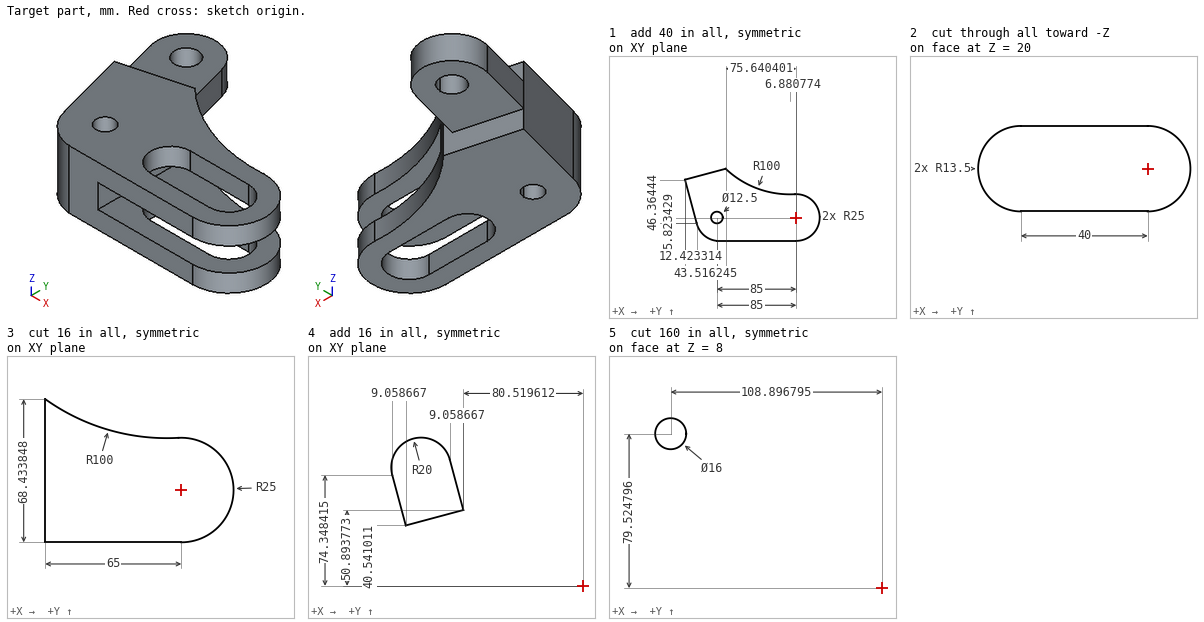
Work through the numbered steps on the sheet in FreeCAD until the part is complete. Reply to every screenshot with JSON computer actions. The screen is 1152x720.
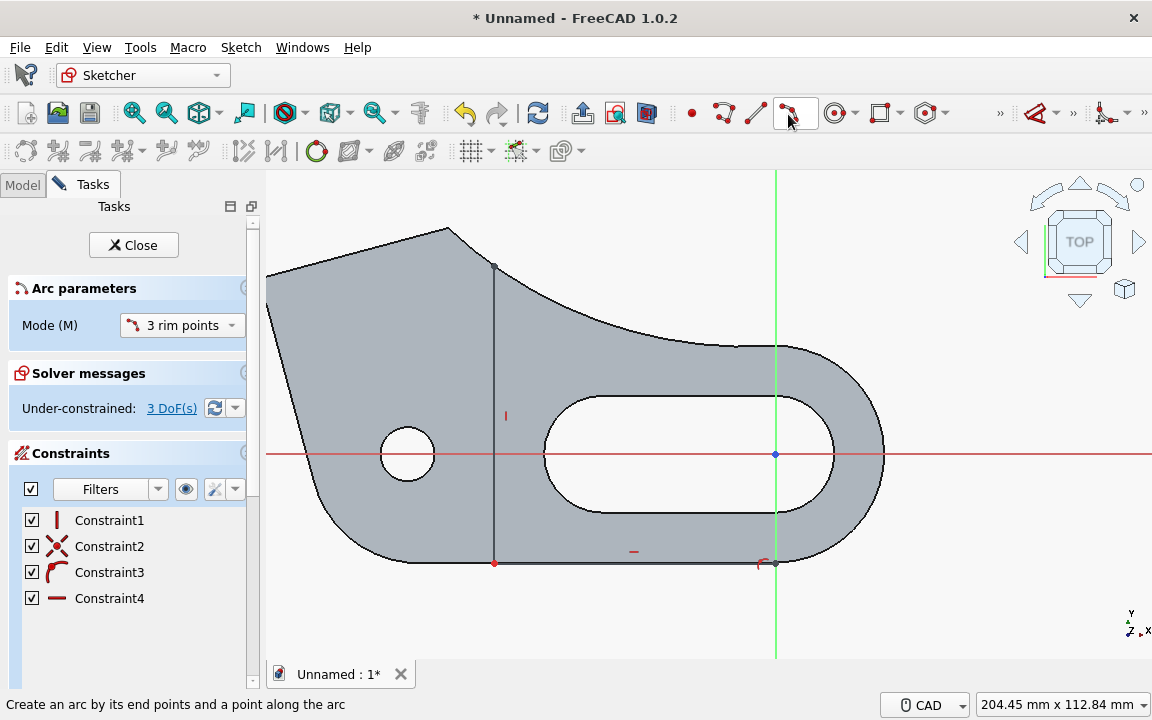
{"action": "left_click", "coordinate": [776, 564]}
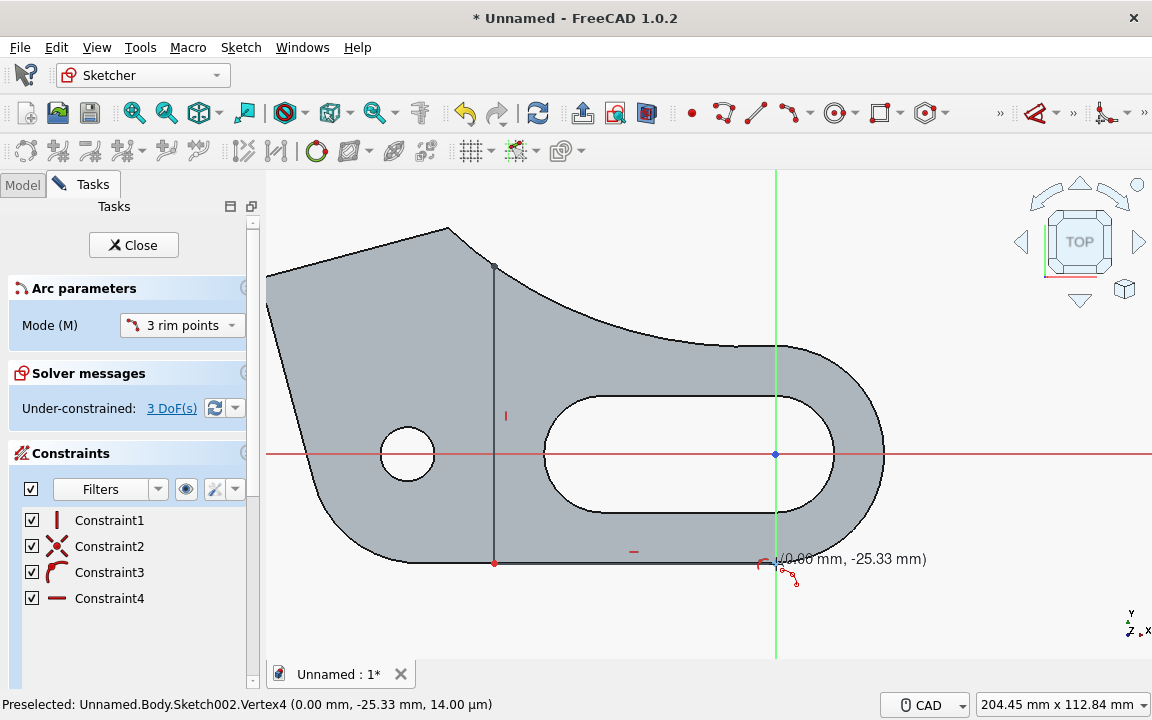
{"action": "scroll", "coordinate": [770, 346], "scroll_direction": "up", "scroll_amount": 5}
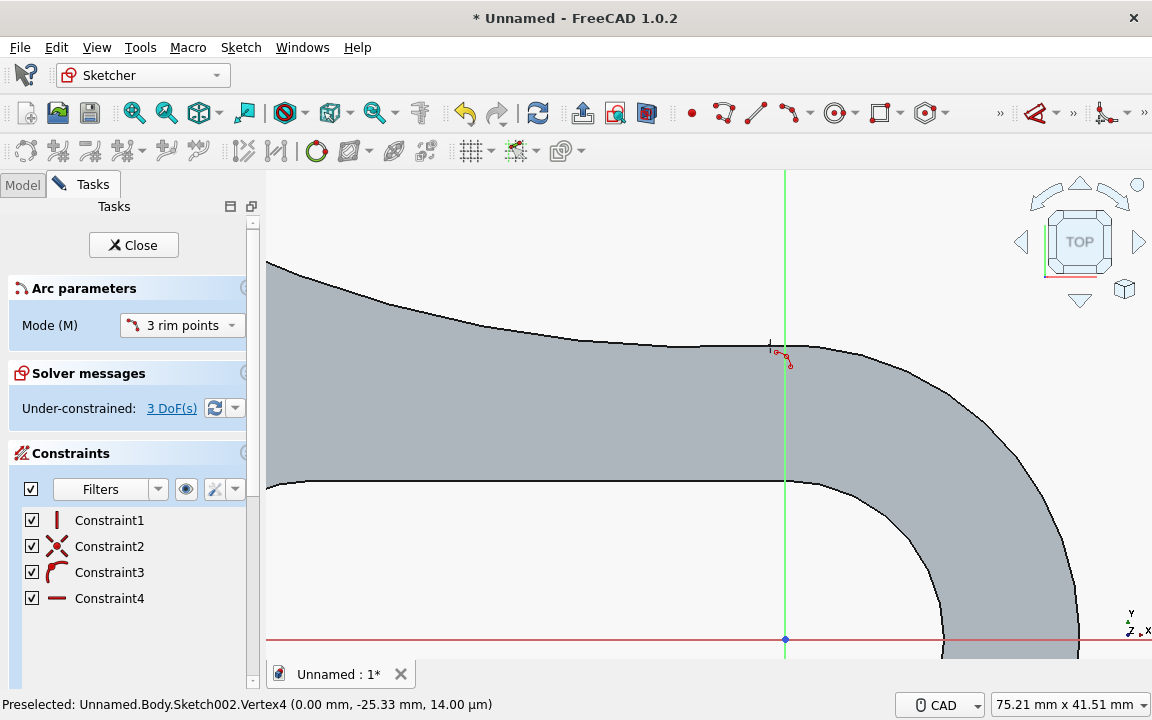
{"action": "left_click", "coordinate": [769, 346]}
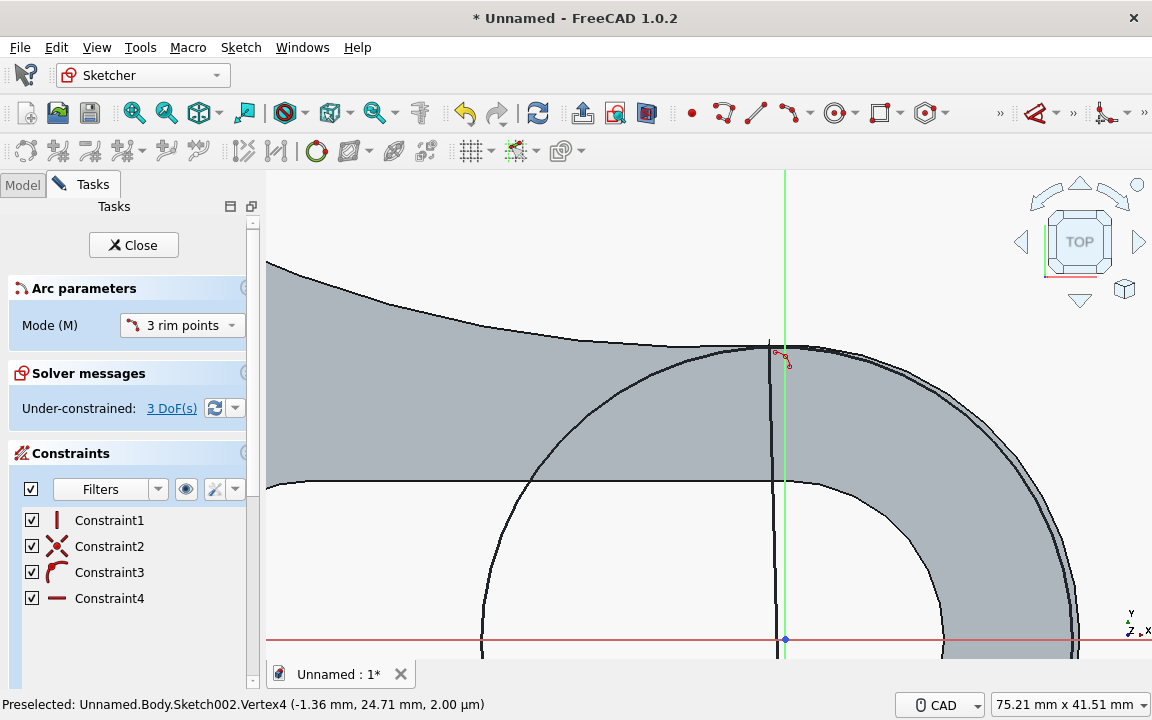
{"action": "scroll", "coordinate": [694, 347], "scroll_direction": "down", "scroll_amount": 5}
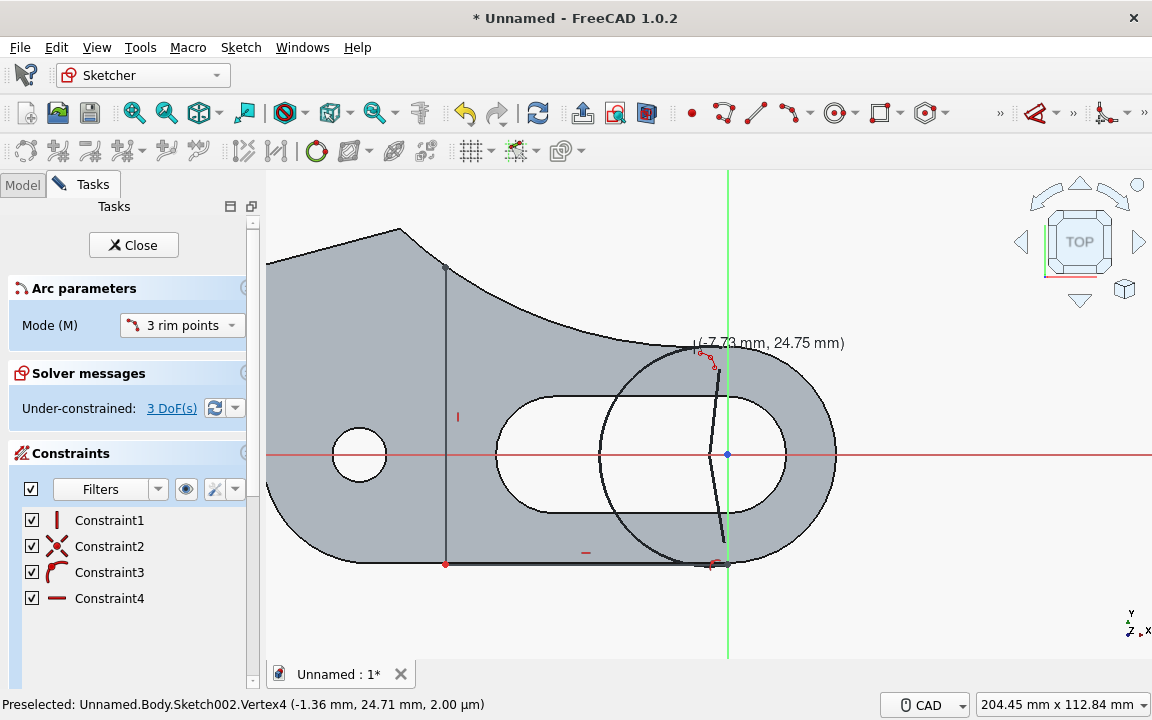
{"action": "left_click", "coordinate": [832, 486]}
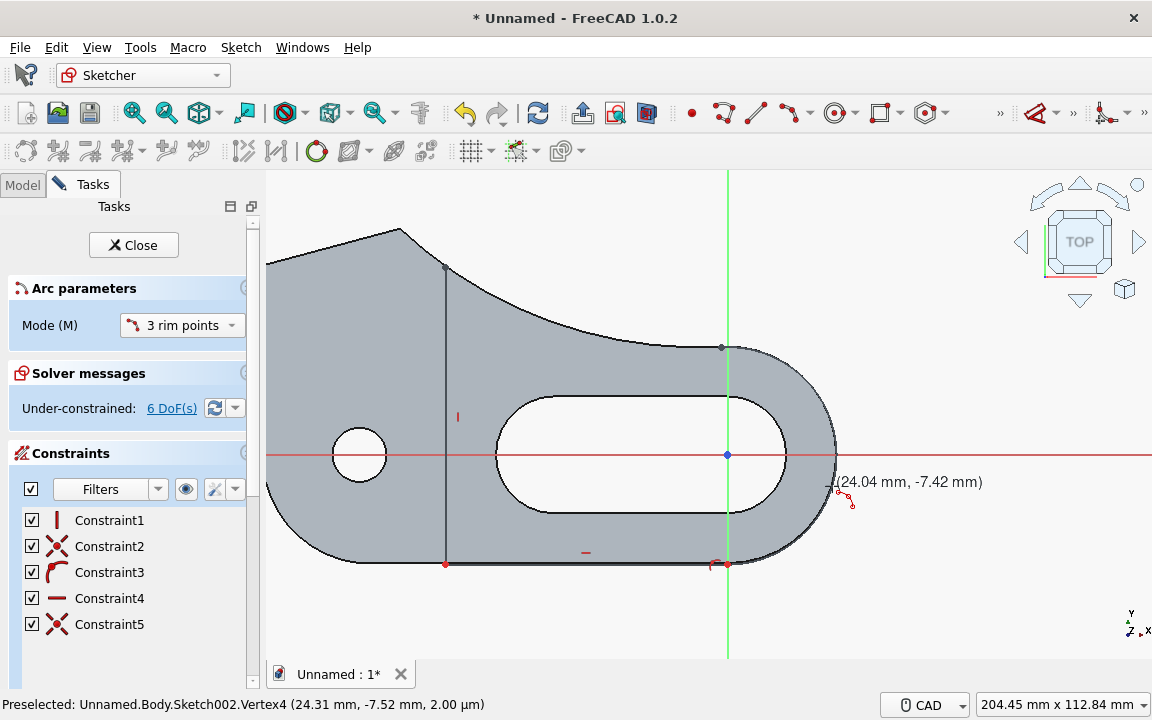
{"action": "scroll", "coordinate": [722, 347], "scroll_direction": "up", "scroll_amount": 5}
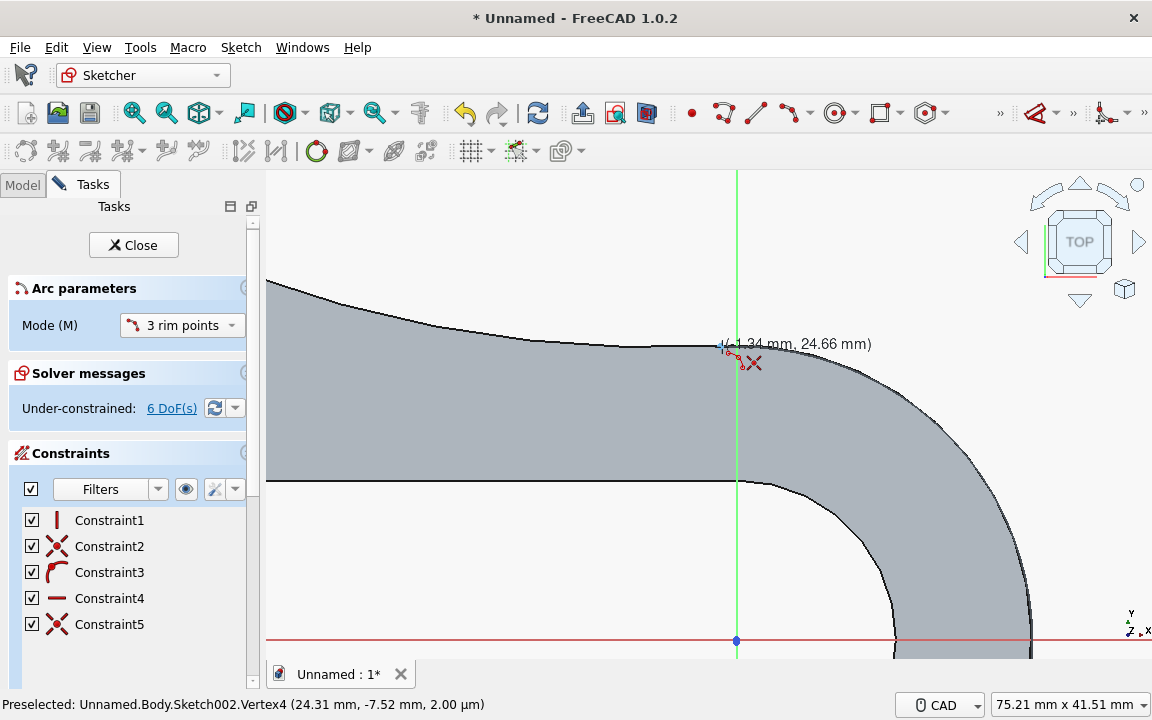
{"action": "left_click", "coordinate": [721, 347]}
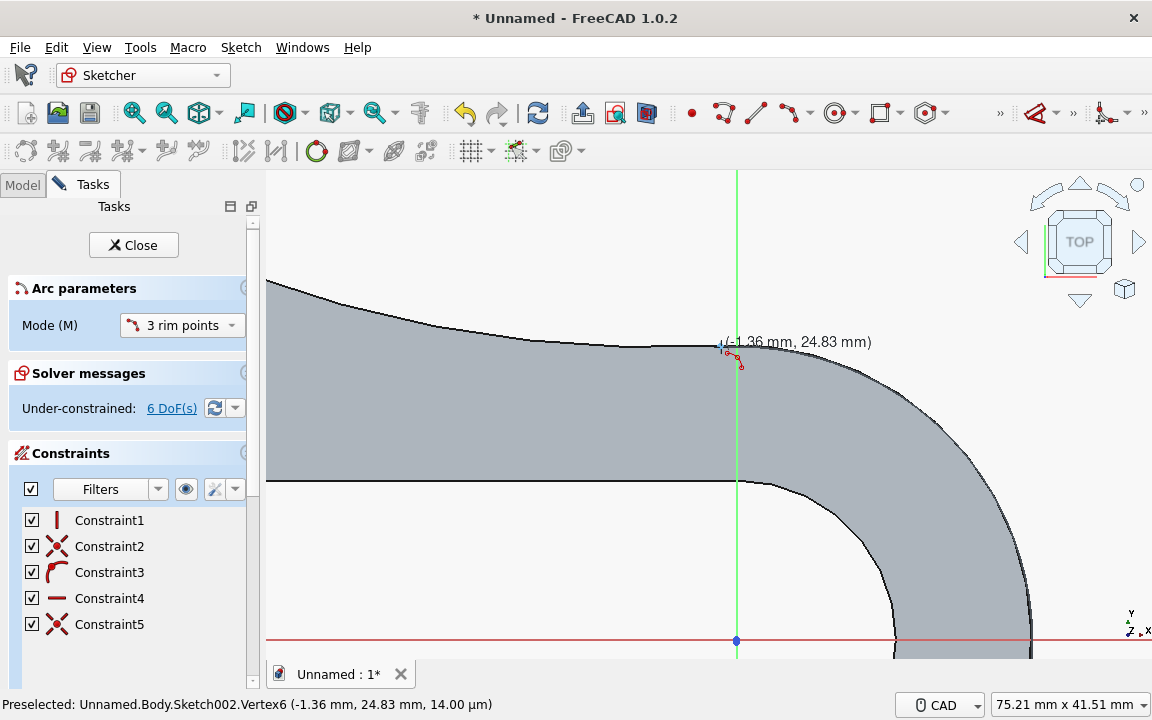
{"action": "scroll", "coordinate": [722, 347], "scroll_direction": "down", "scroll_amount": 5}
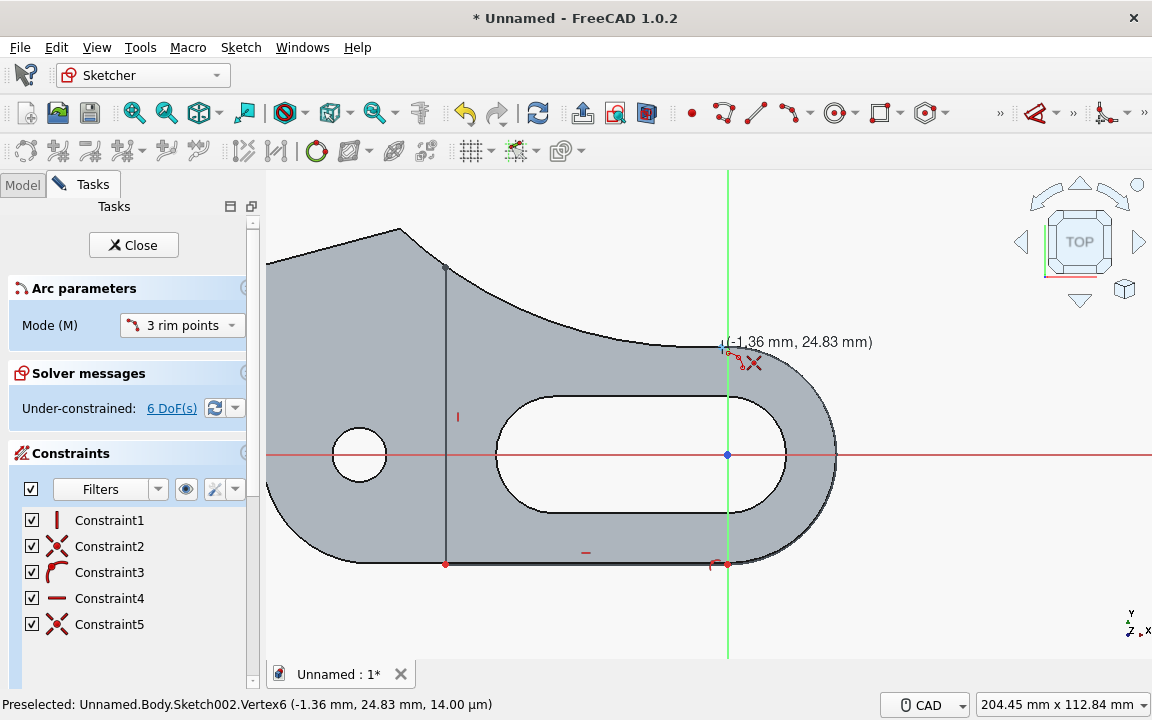
{"action": "left_click", "coordinate": [446, 268]}
{"action": "left_click", "coordinate": [577, 330]}
{"action": "key", "text": "Escape"}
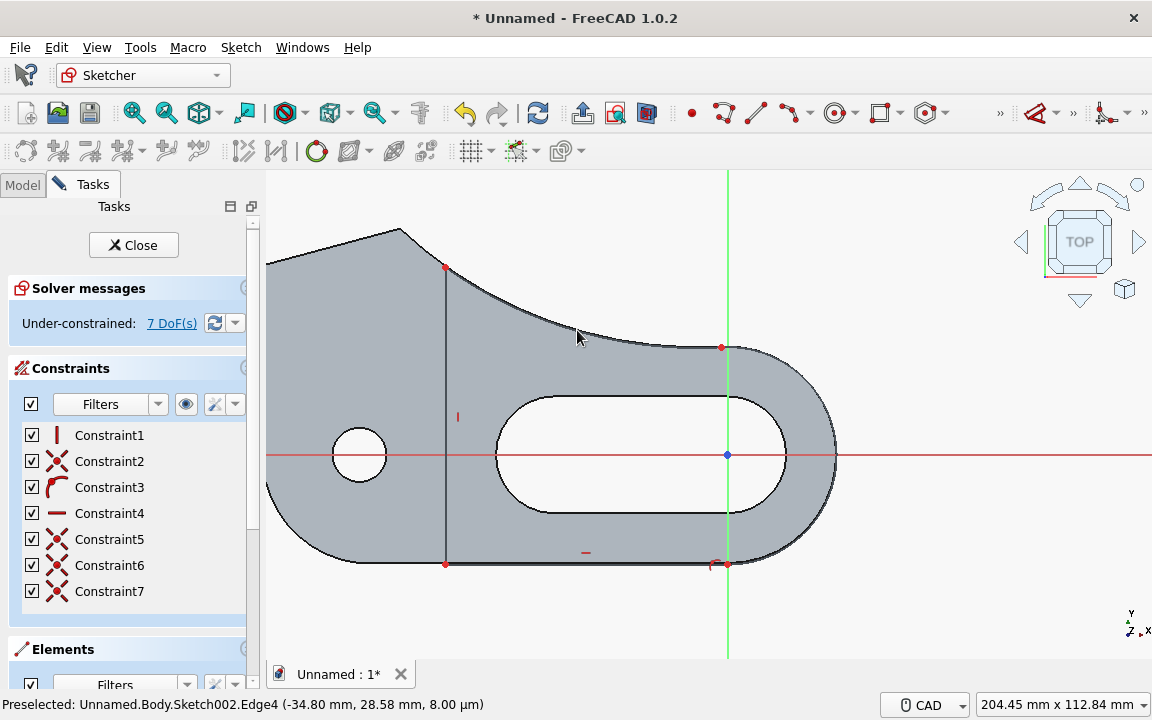
{"action": "left_click", "coordinate": [530, 565]}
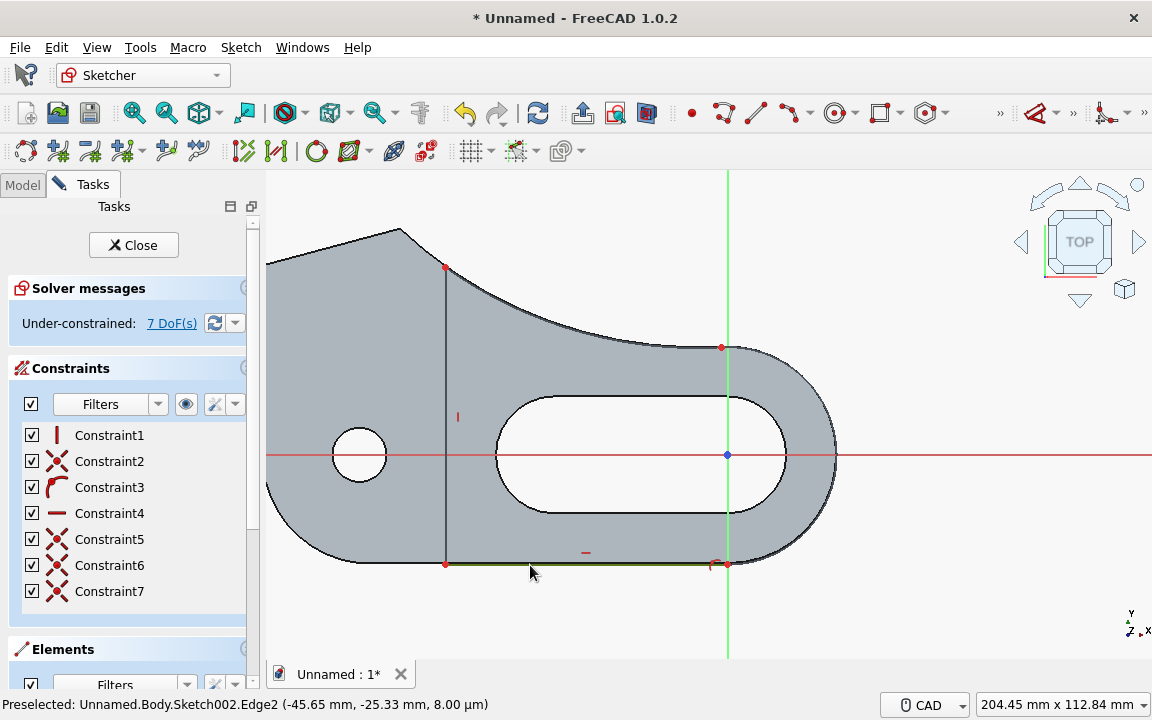
{"action": "left_click", "coordinate": [817, 518]}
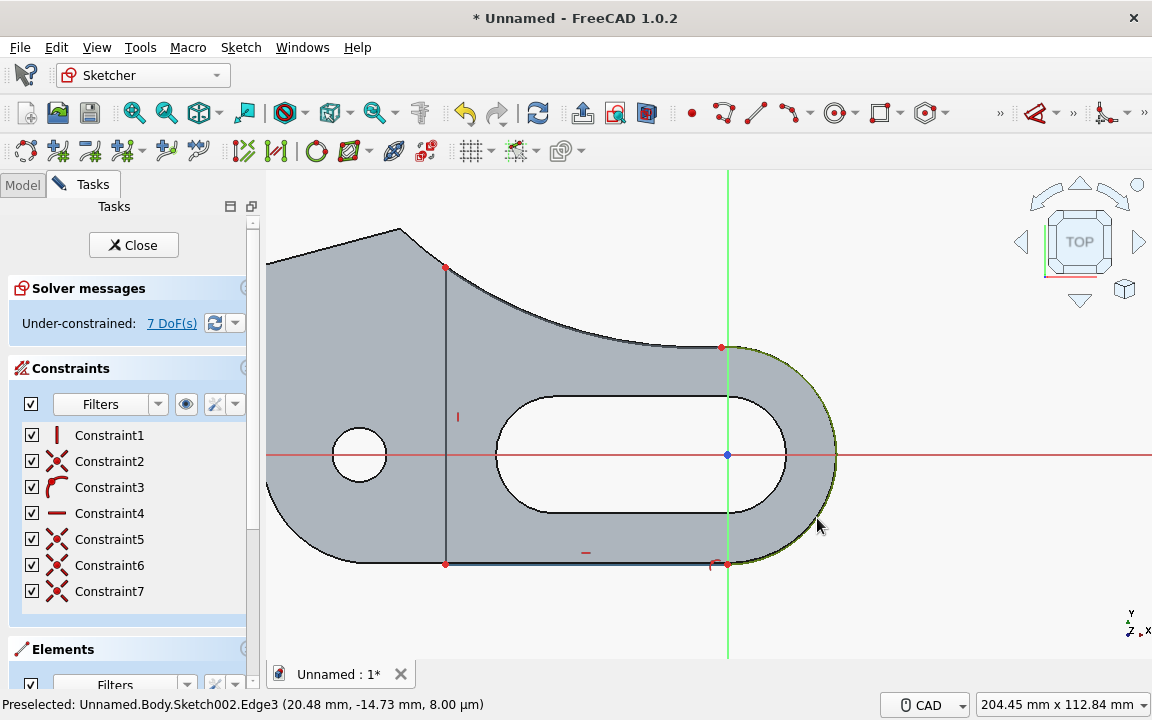
{"action": "key", "text": "t"}